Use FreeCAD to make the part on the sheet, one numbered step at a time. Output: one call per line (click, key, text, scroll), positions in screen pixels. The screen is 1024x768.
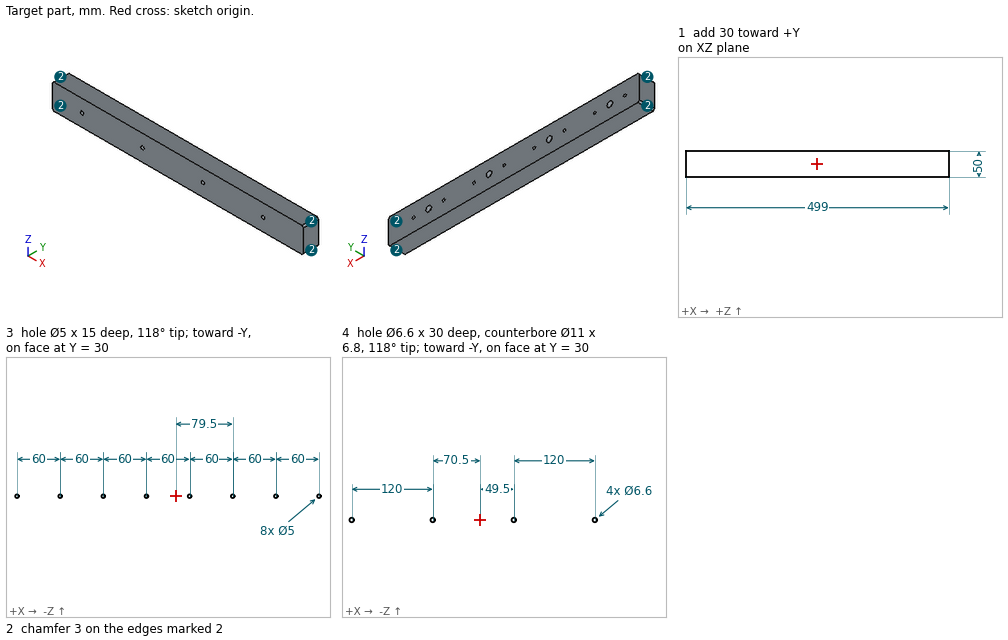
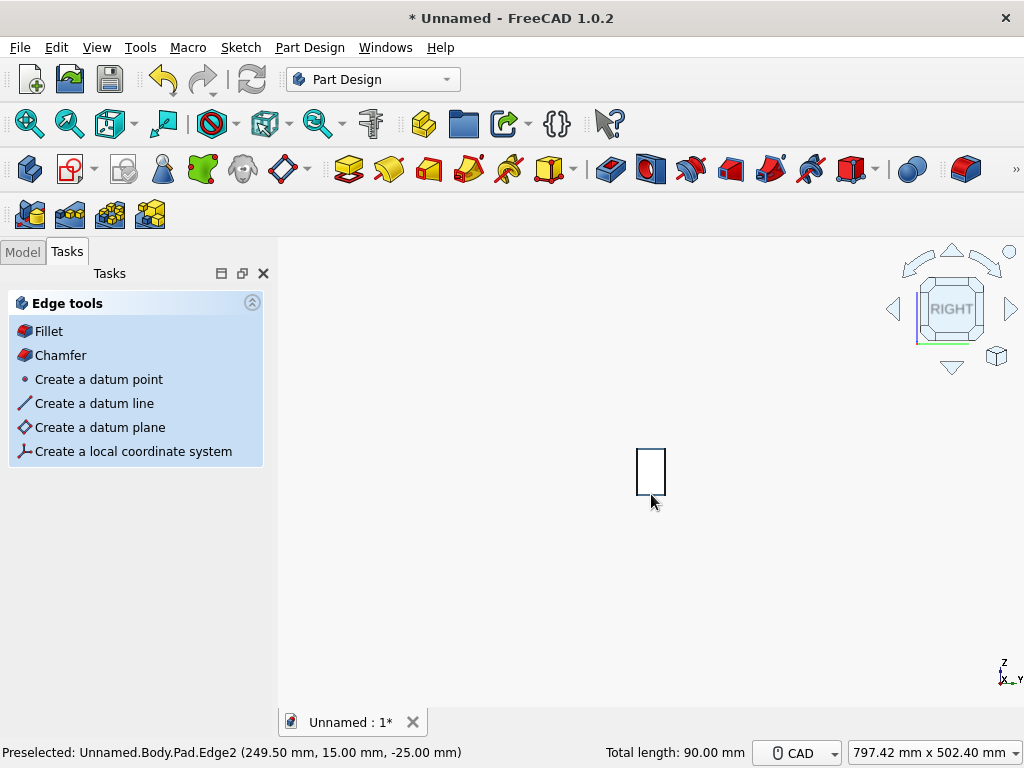
key(5)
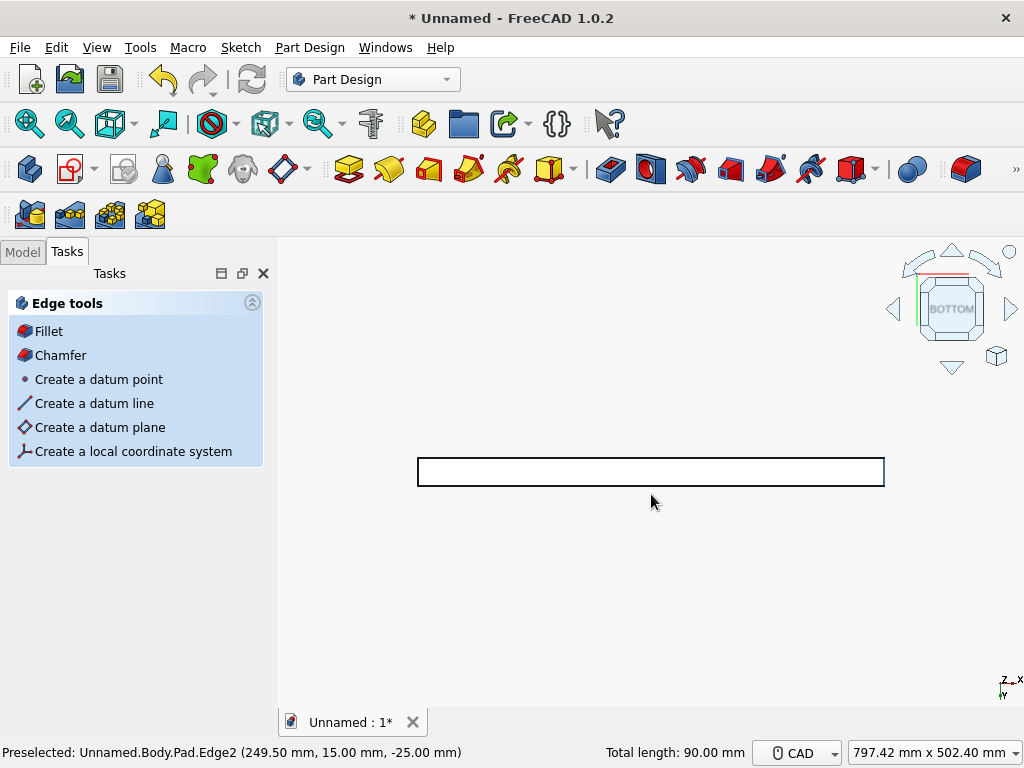
click(418, 471, ctrl)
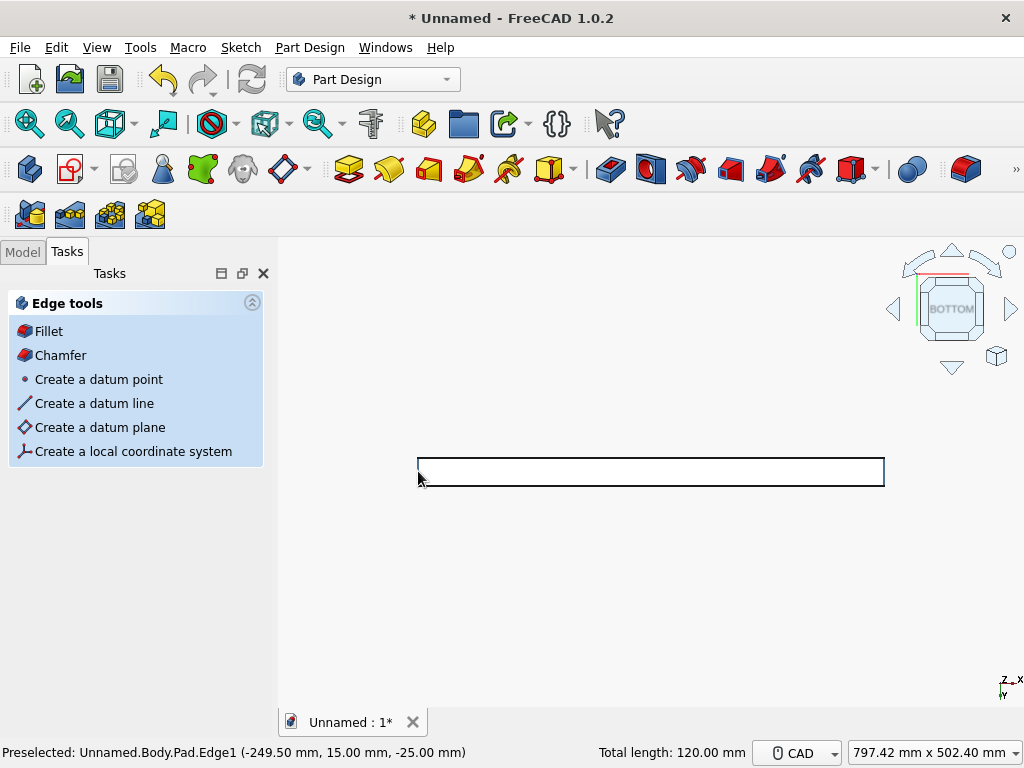
click(136, 355)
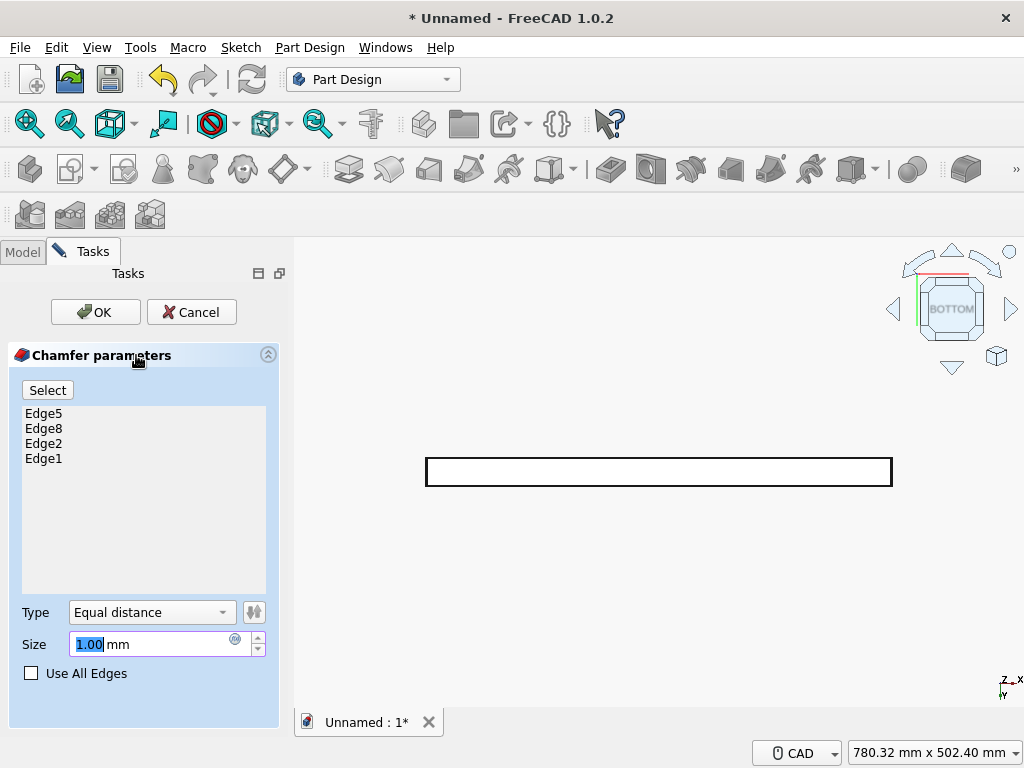
text(3)
key(Tab)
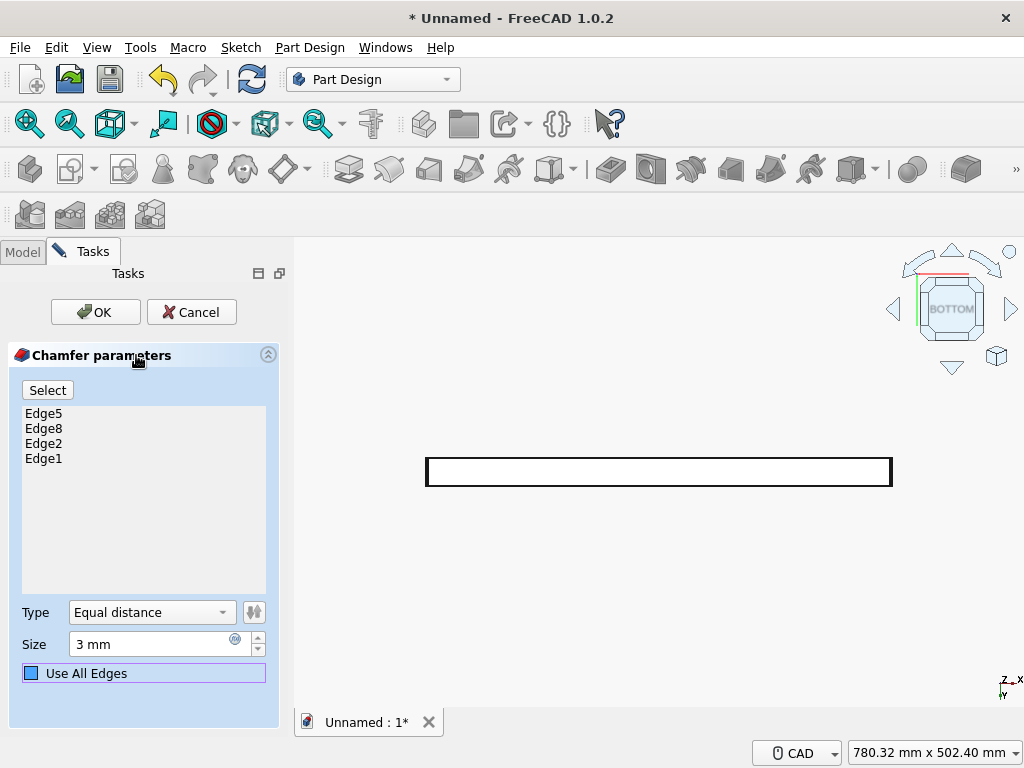
click(96, 312)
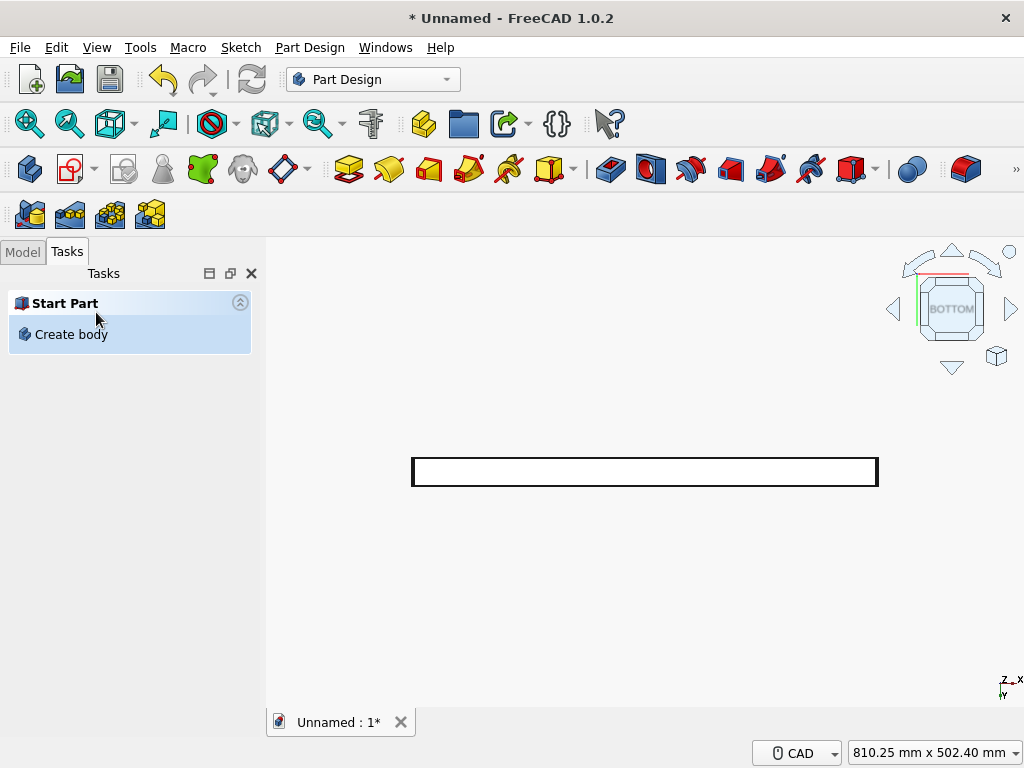
key(4)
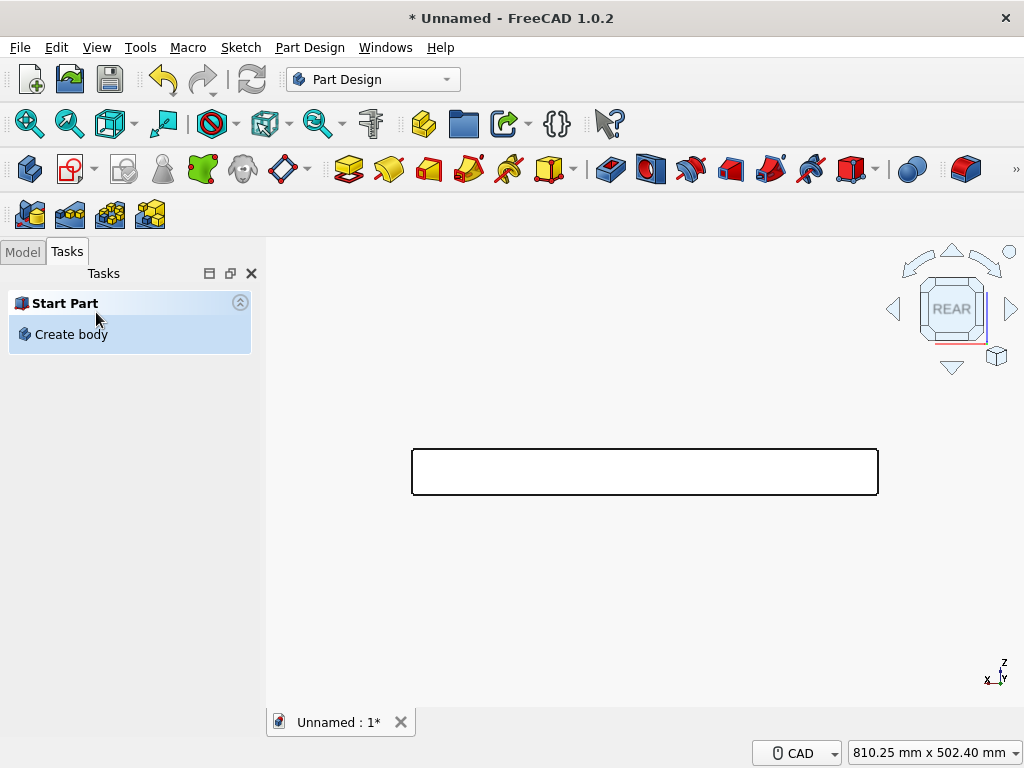
click(445, 471)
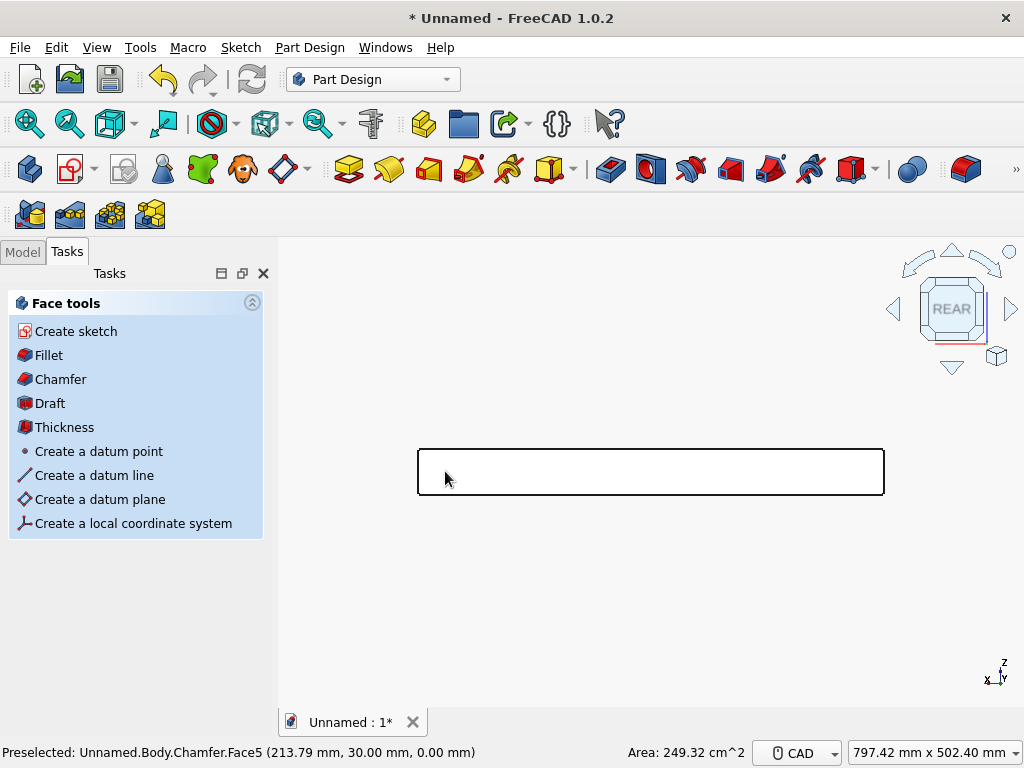
click(70, 170)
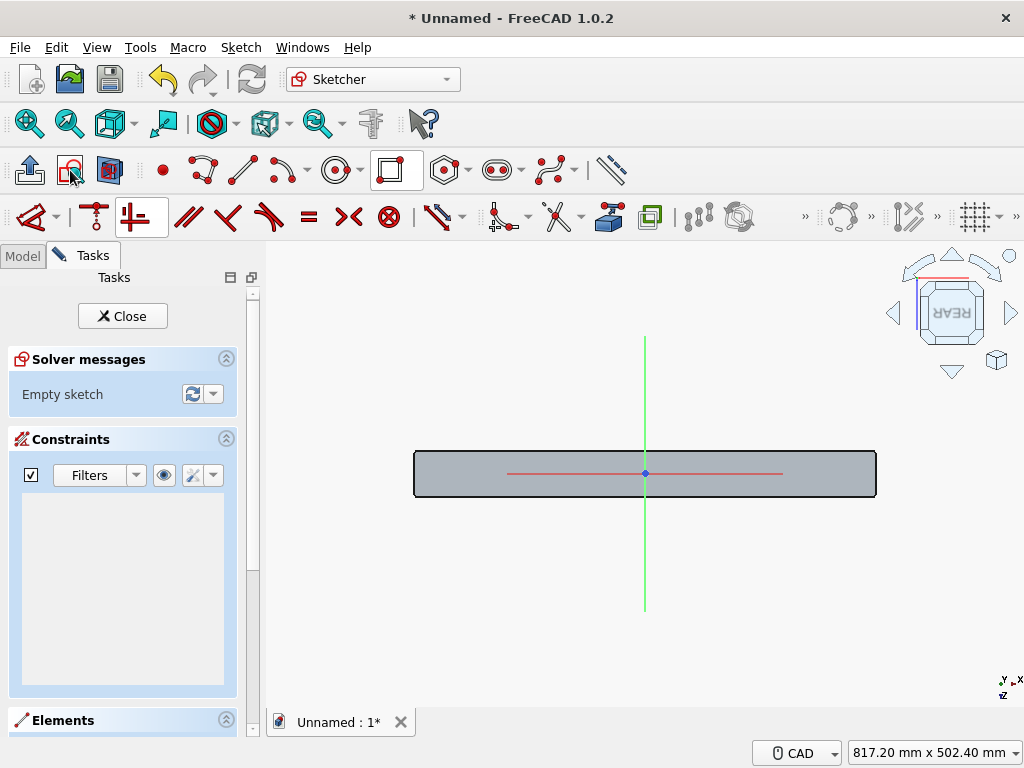
click(336, 170)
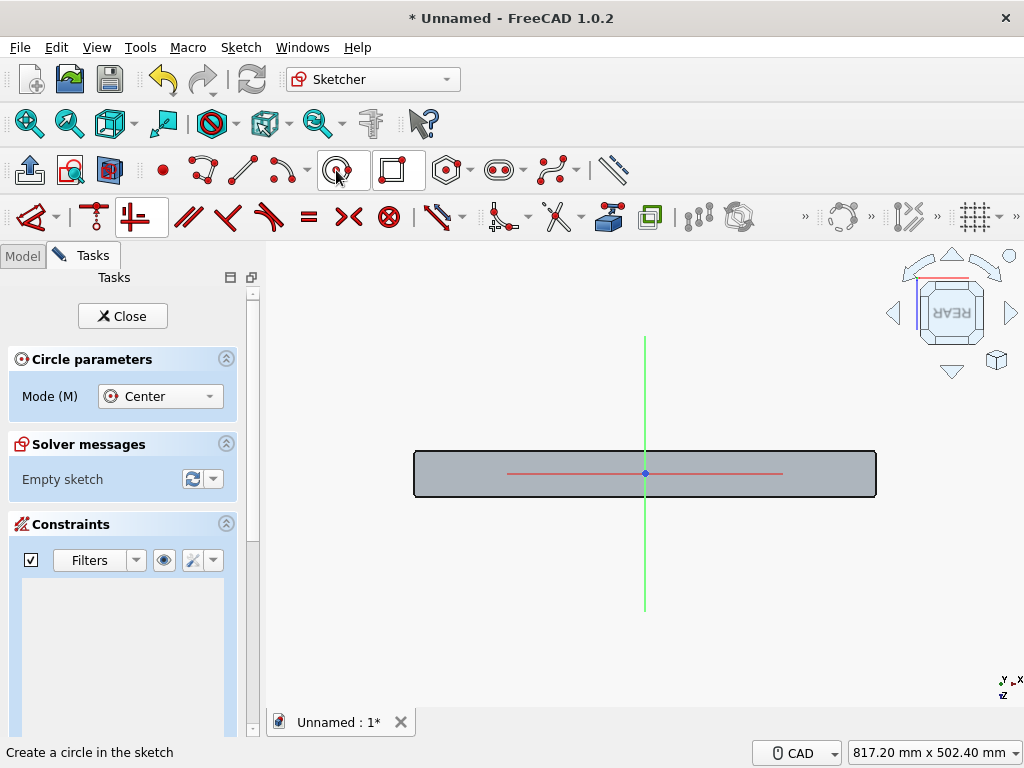
scroll(830, 474, up, 12)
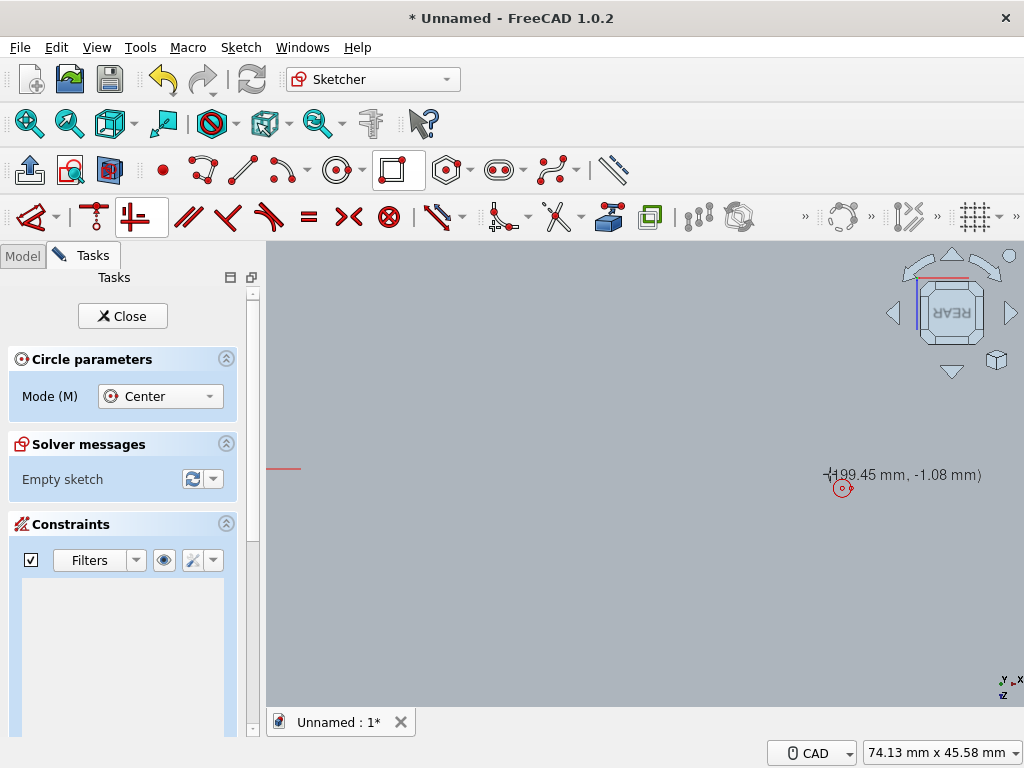
scroll(766, 475, down, 12)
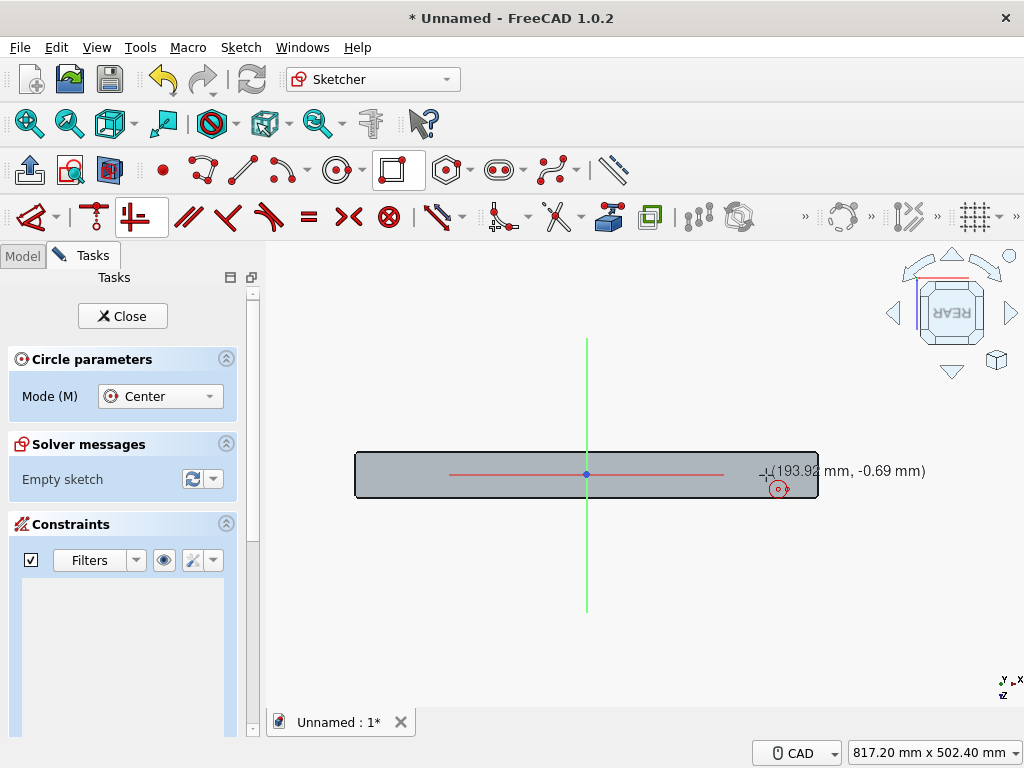
click(772, 475)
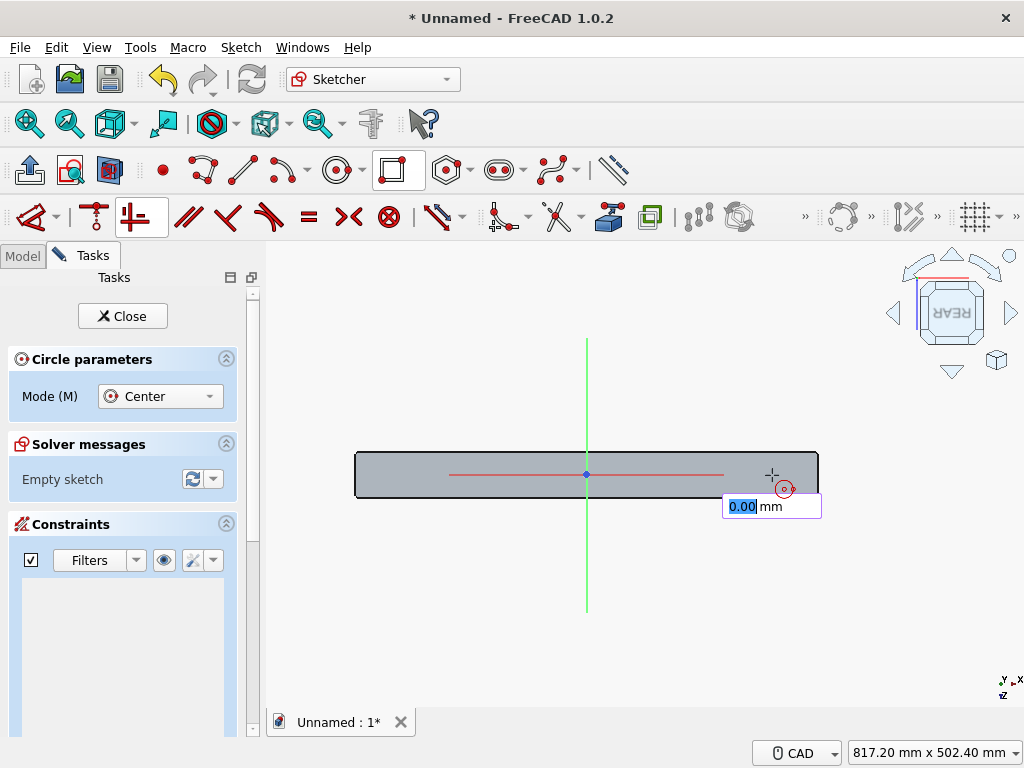
scroll(771, 477, up, 10)